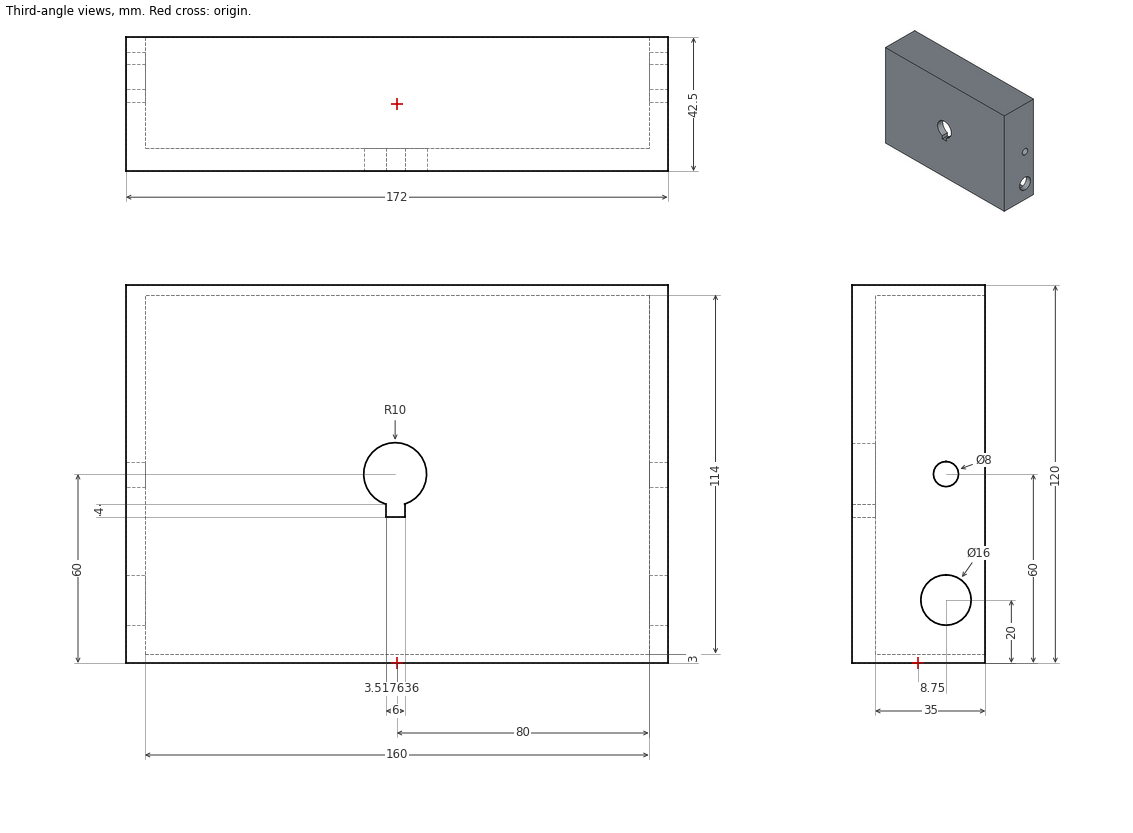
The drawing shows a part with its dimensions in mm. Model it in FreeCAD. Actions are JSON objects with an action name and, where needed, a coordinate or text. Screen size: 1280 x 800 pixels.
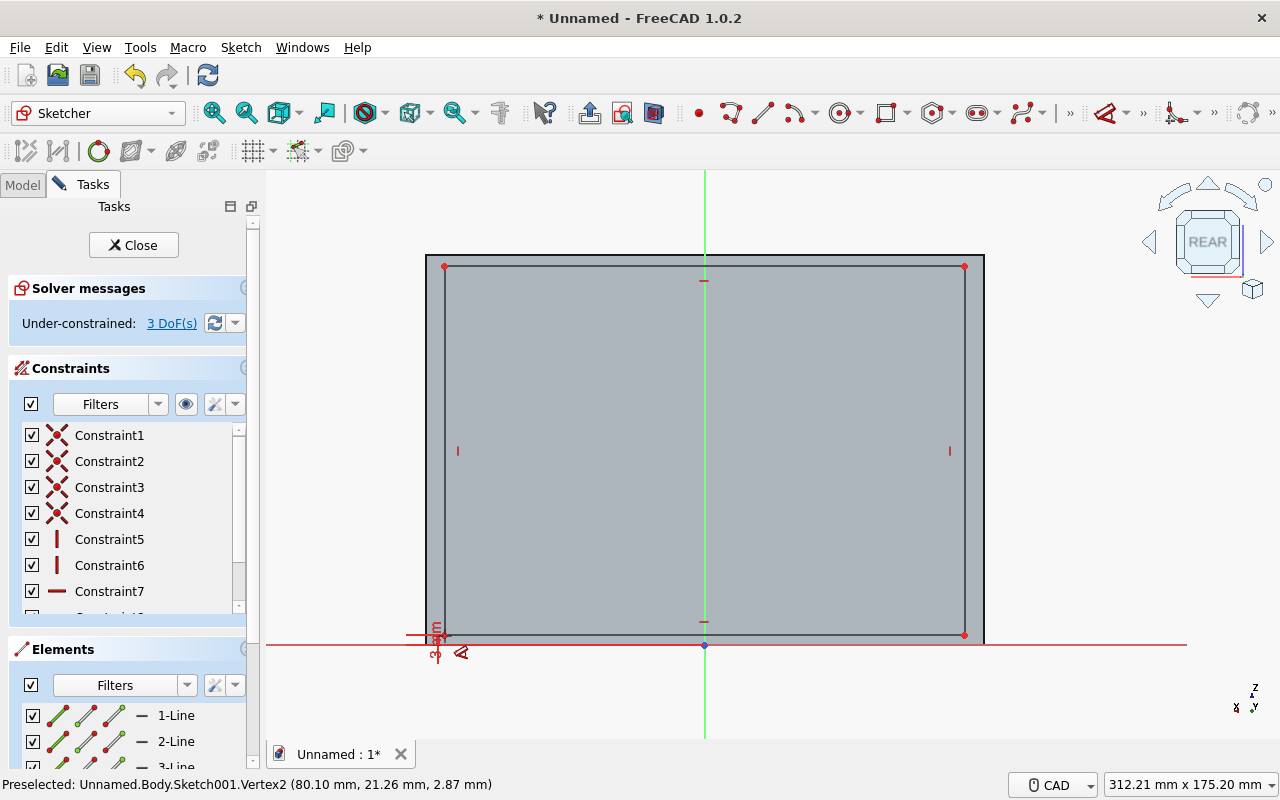
{"action": "left_click", "coordinate": [445, 562]}
{"action": "left_click", "coordinate": [411, 451]}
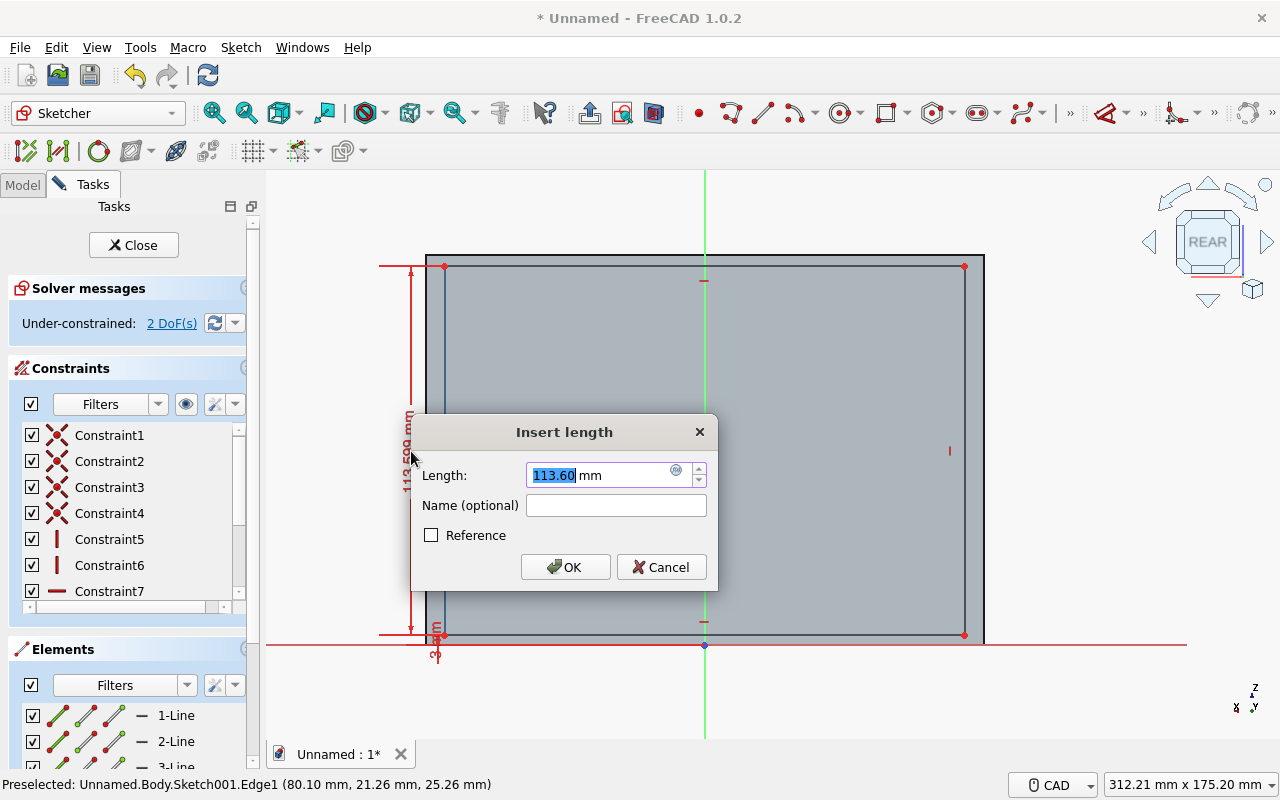
{"action": "type", "text": "114"}
{"action": "key", "text": "Return"}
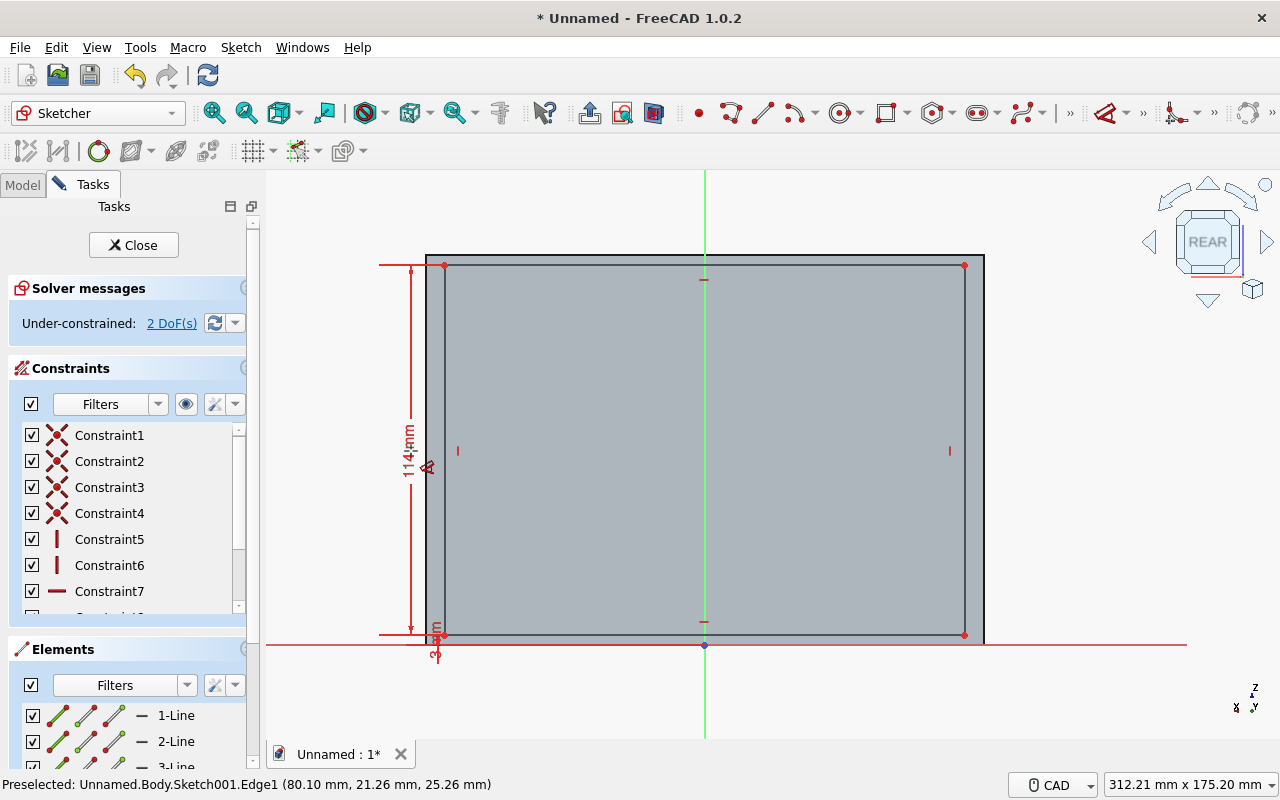
{"action": "scroll", "coordinate": [601, 635], "scroll_direction": "up", "scroll_amount": 2}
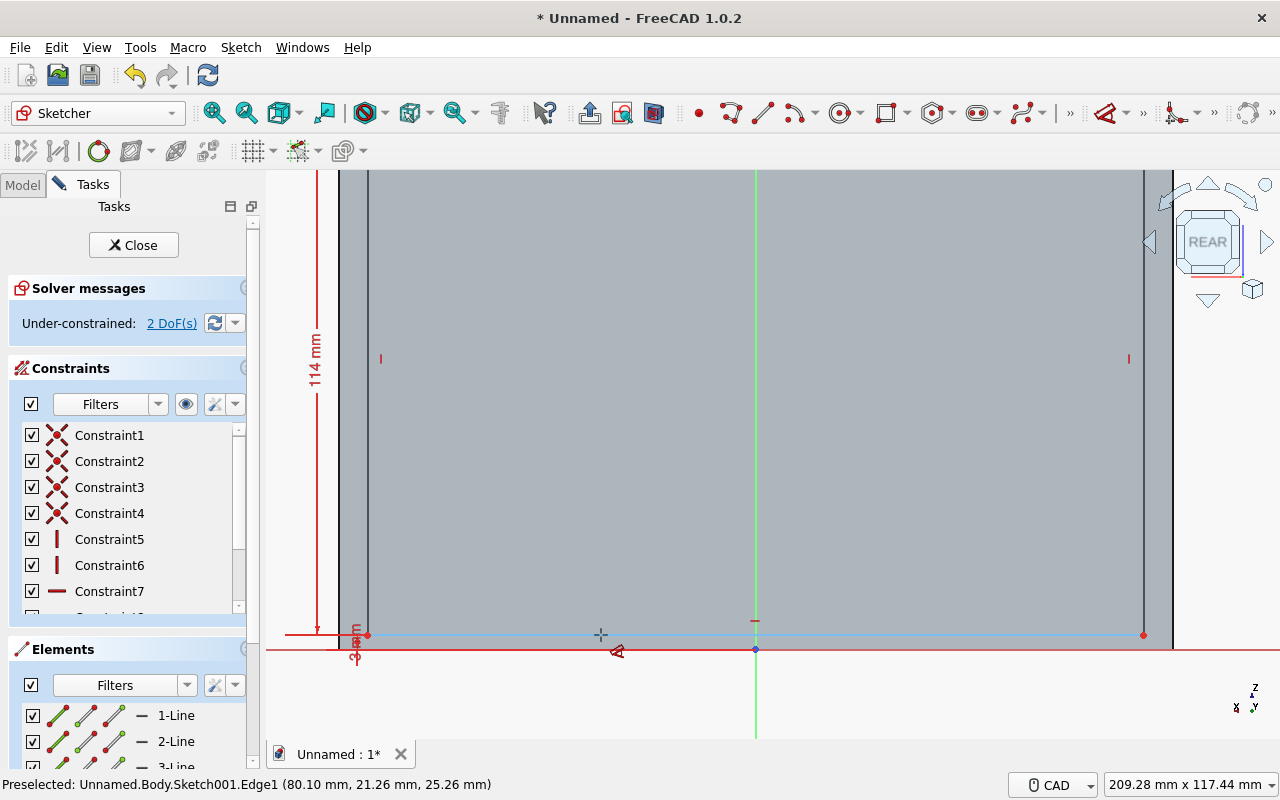
{"action": "left_click", "coordinate": [601, 635]}
{"action": "left_click", "coordinate": [741, 669]}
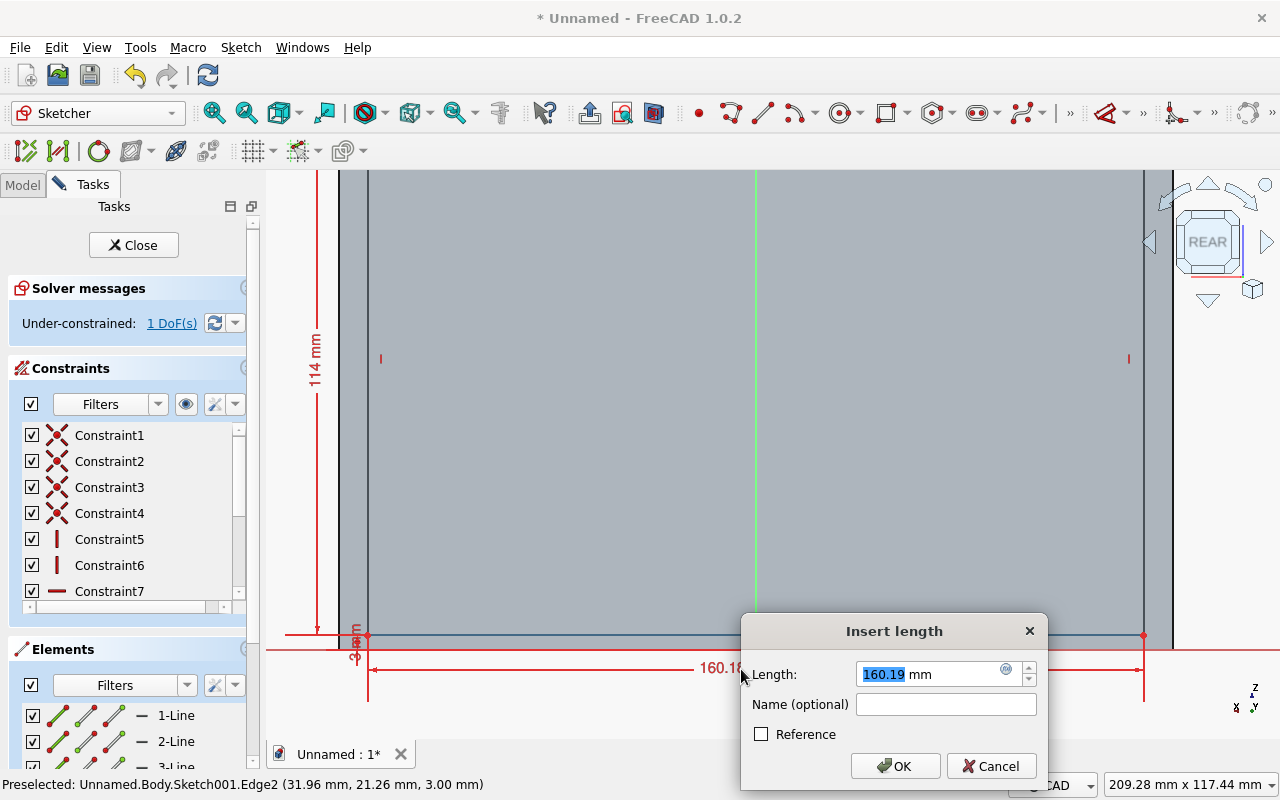
{"action": "type", "text": "160"}
{"action": "key", "text": "Return"}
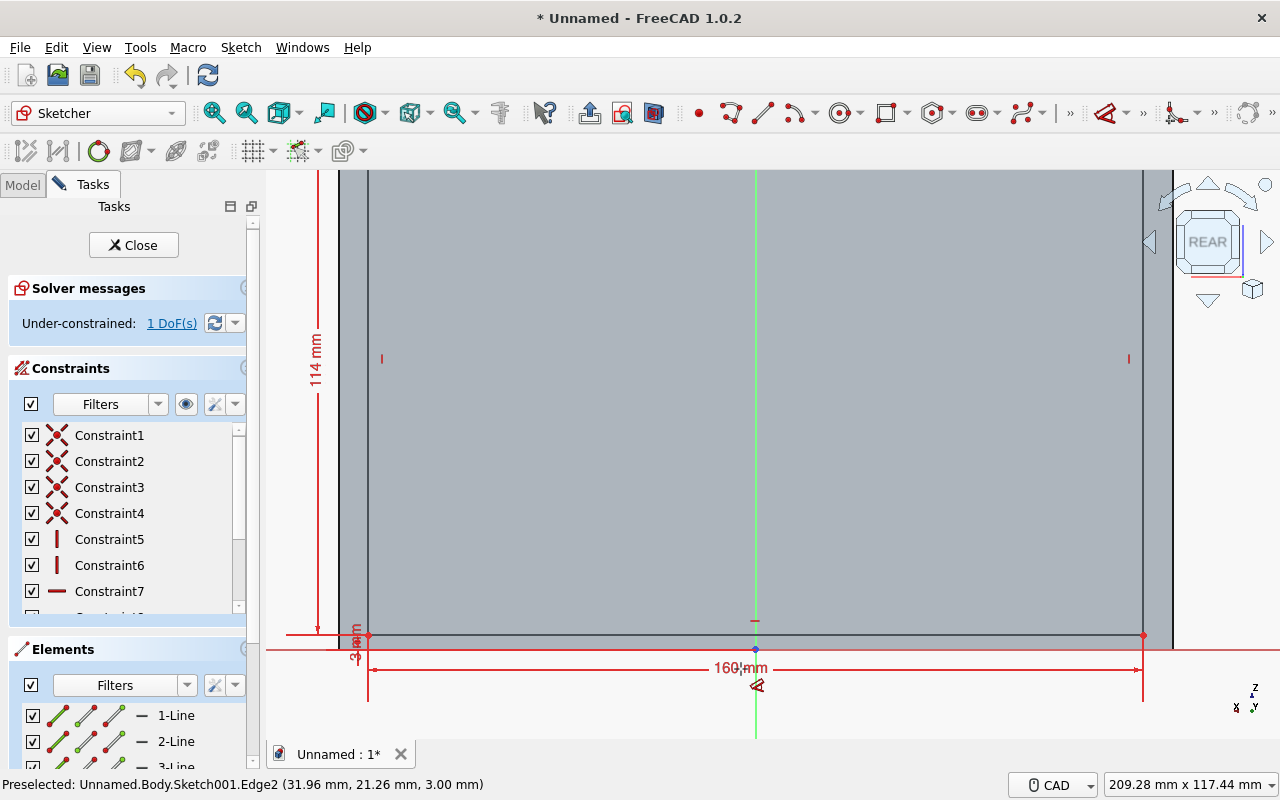
{"action": "scroll", "coordinate": [600, 634], "scroll_direction": "down", "scroll_amount": 2}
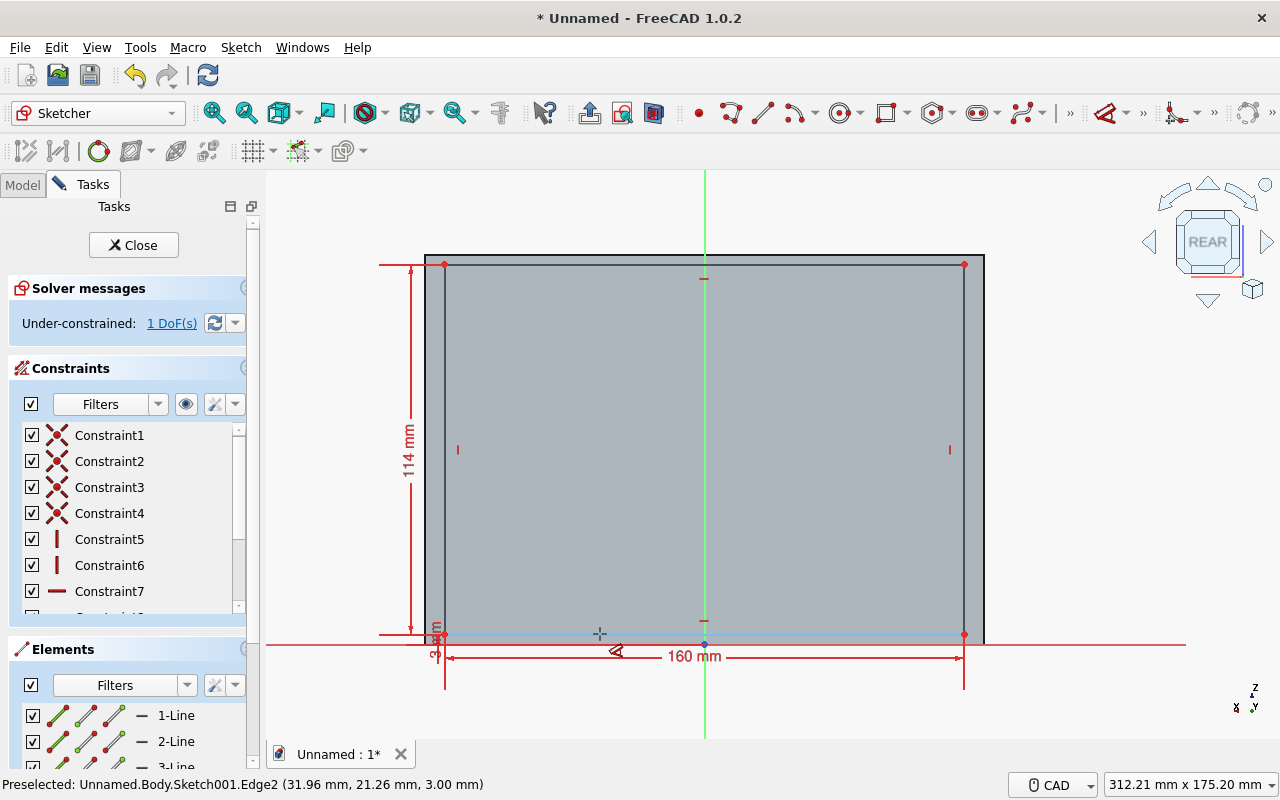
{"action": "left_click", "coordinate": [445, 265]}
{"action": "left_click", "coordinate": [575, 679]}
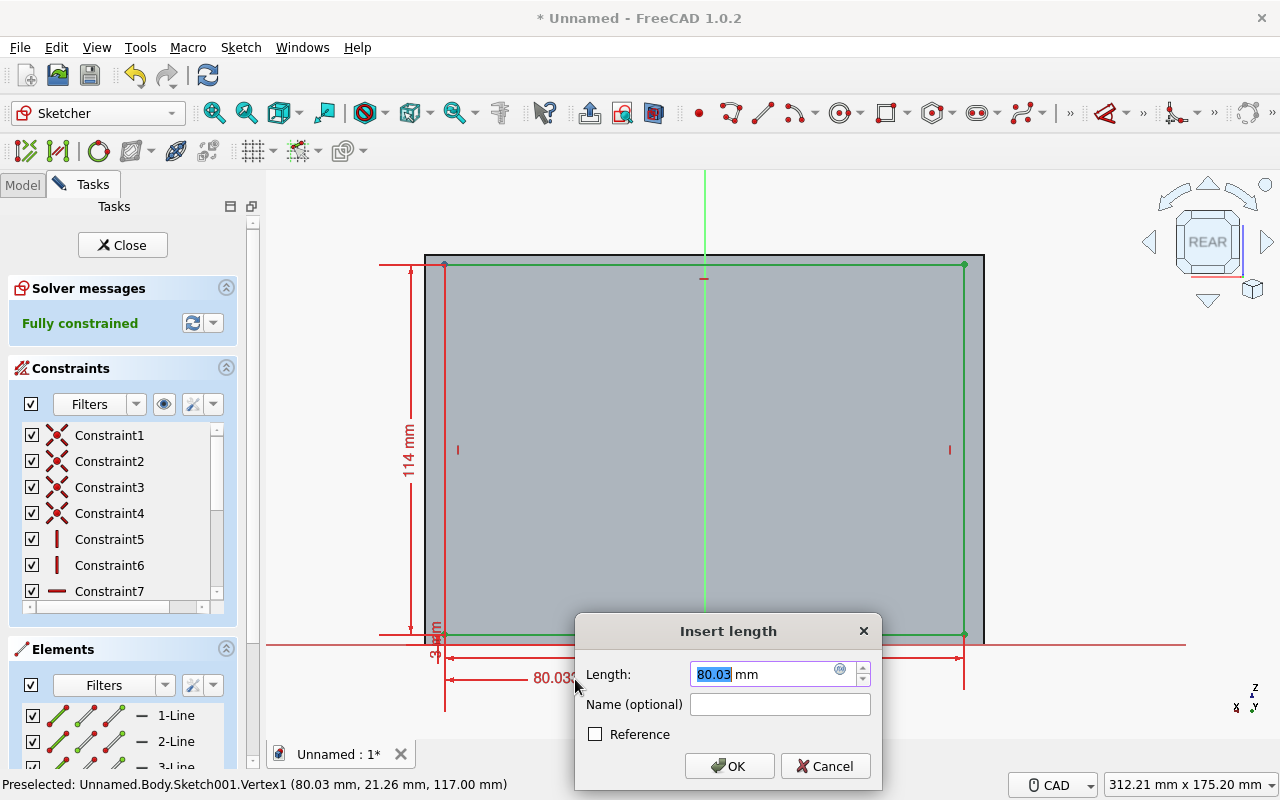
{"action": "type", "text": "80"}
{"action": "key", "text": "Return"}
{"action": "key", "text": "Escape"}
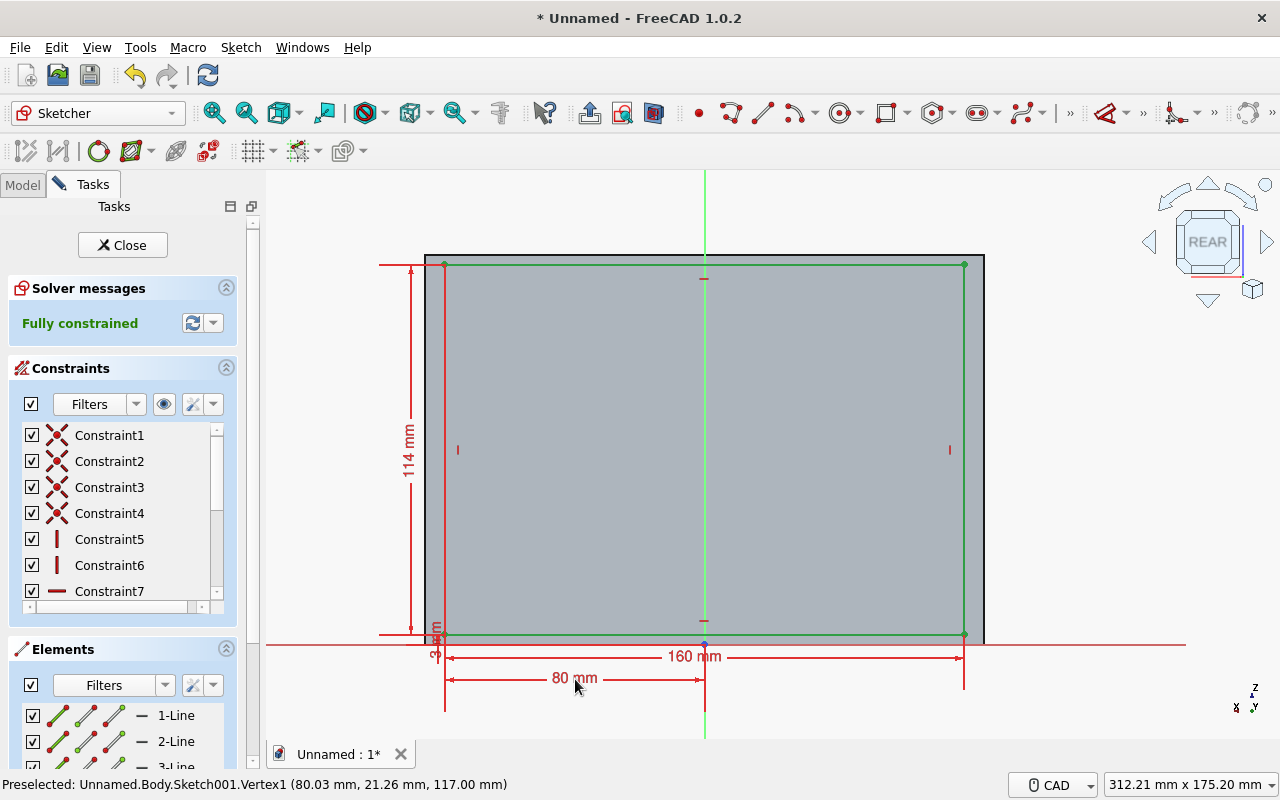
{"action": "left_click", "coordinate": [123, 245]}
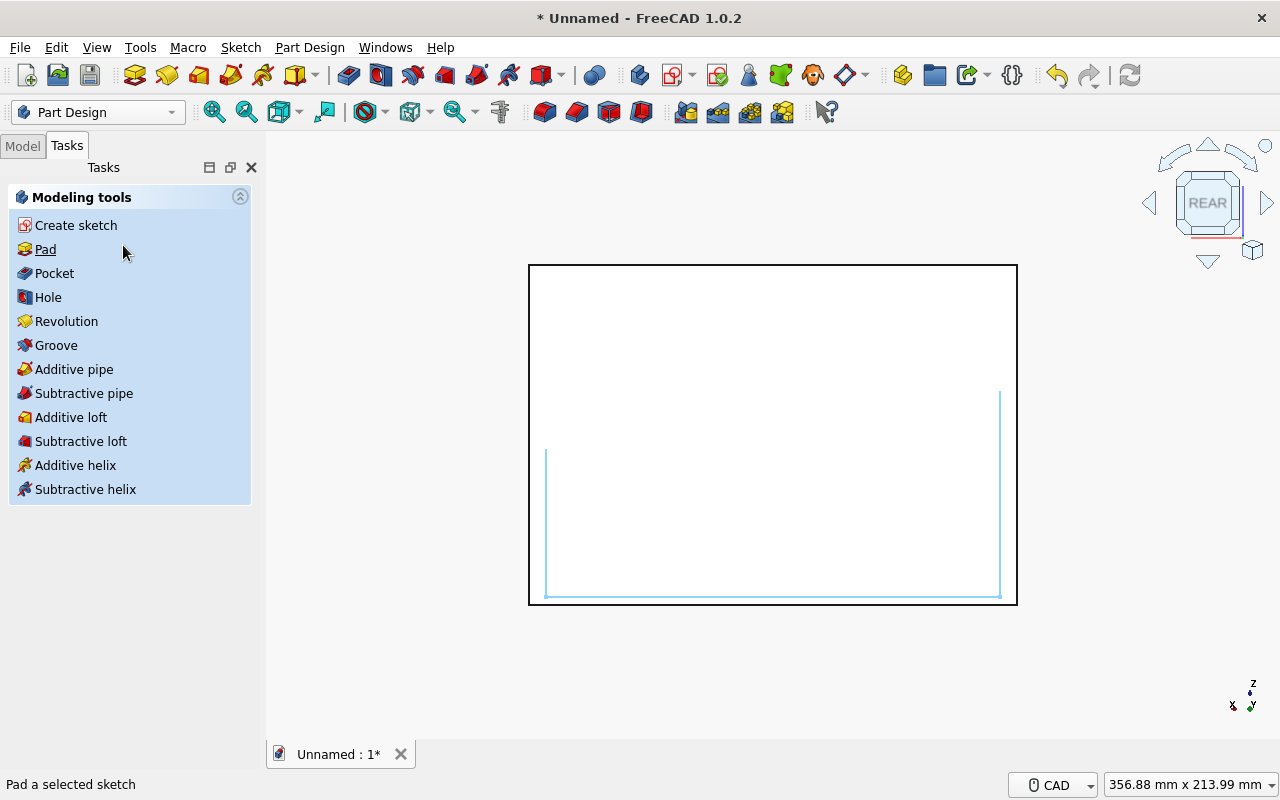
{"action": "left_click", "coordinate": [350, 76]}